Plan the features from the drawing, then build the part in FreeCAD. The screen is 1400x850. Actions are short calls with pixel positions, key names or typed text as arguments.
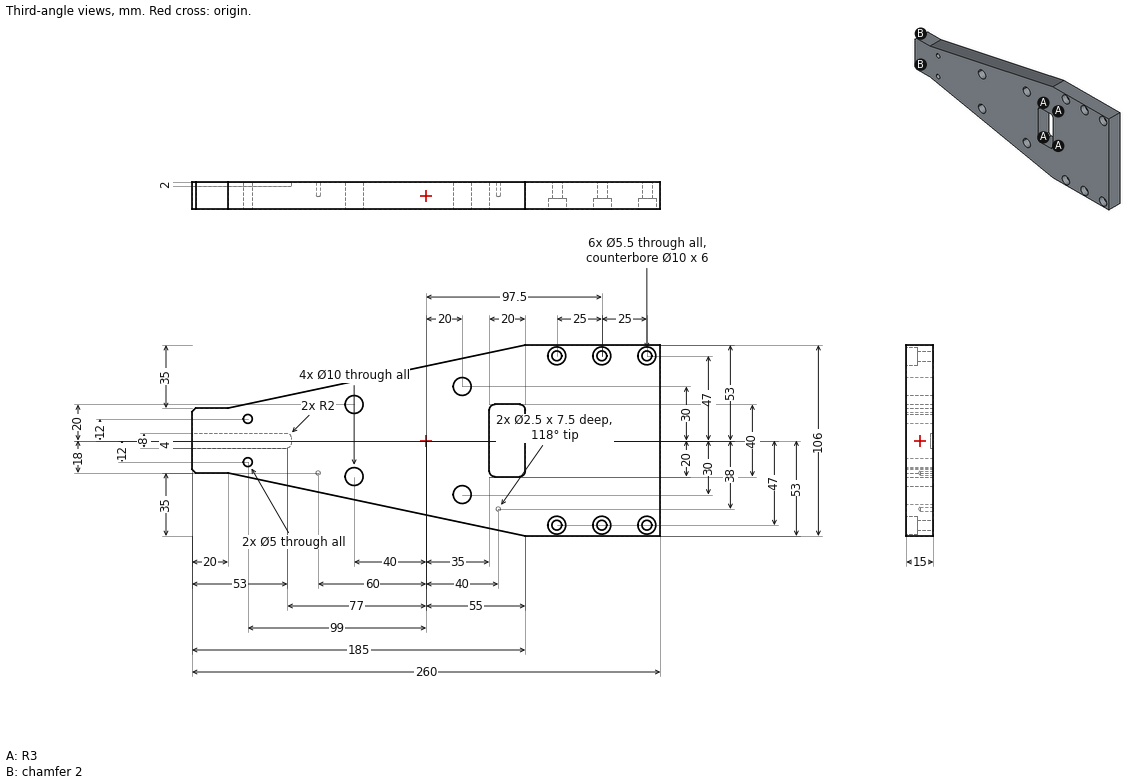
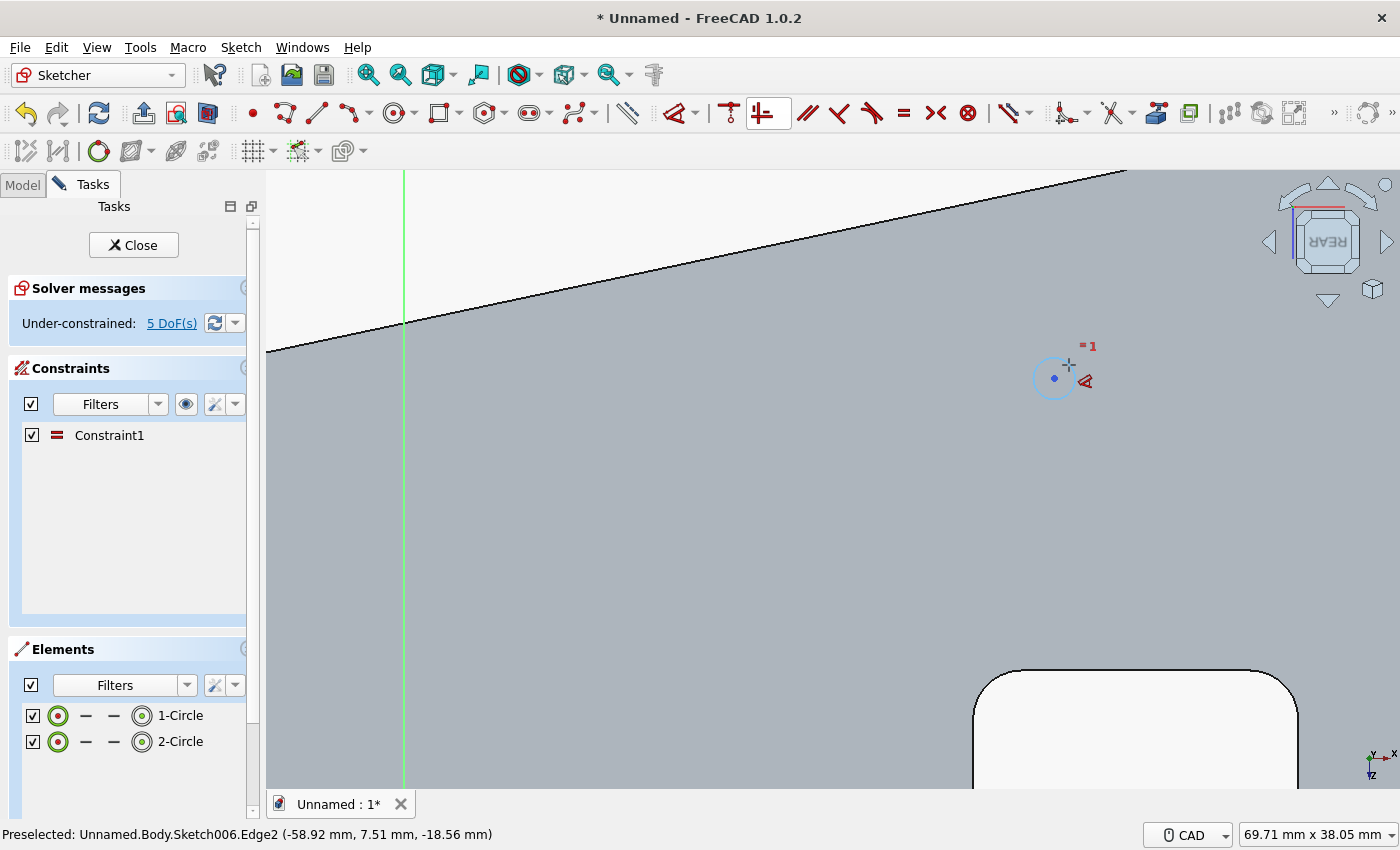
click(1069, 364)
click(1092, 341)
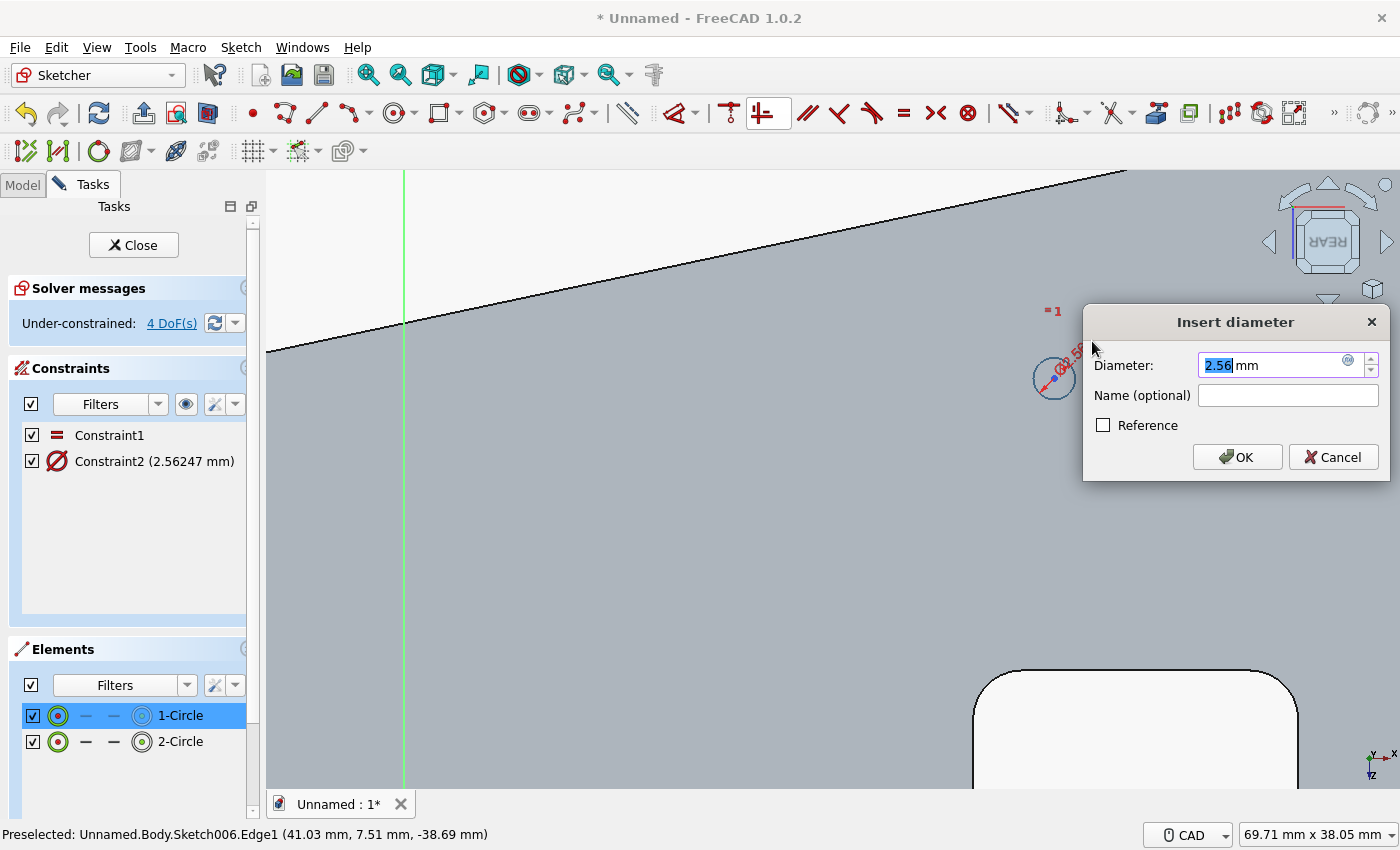
text(2.5)
key(Return)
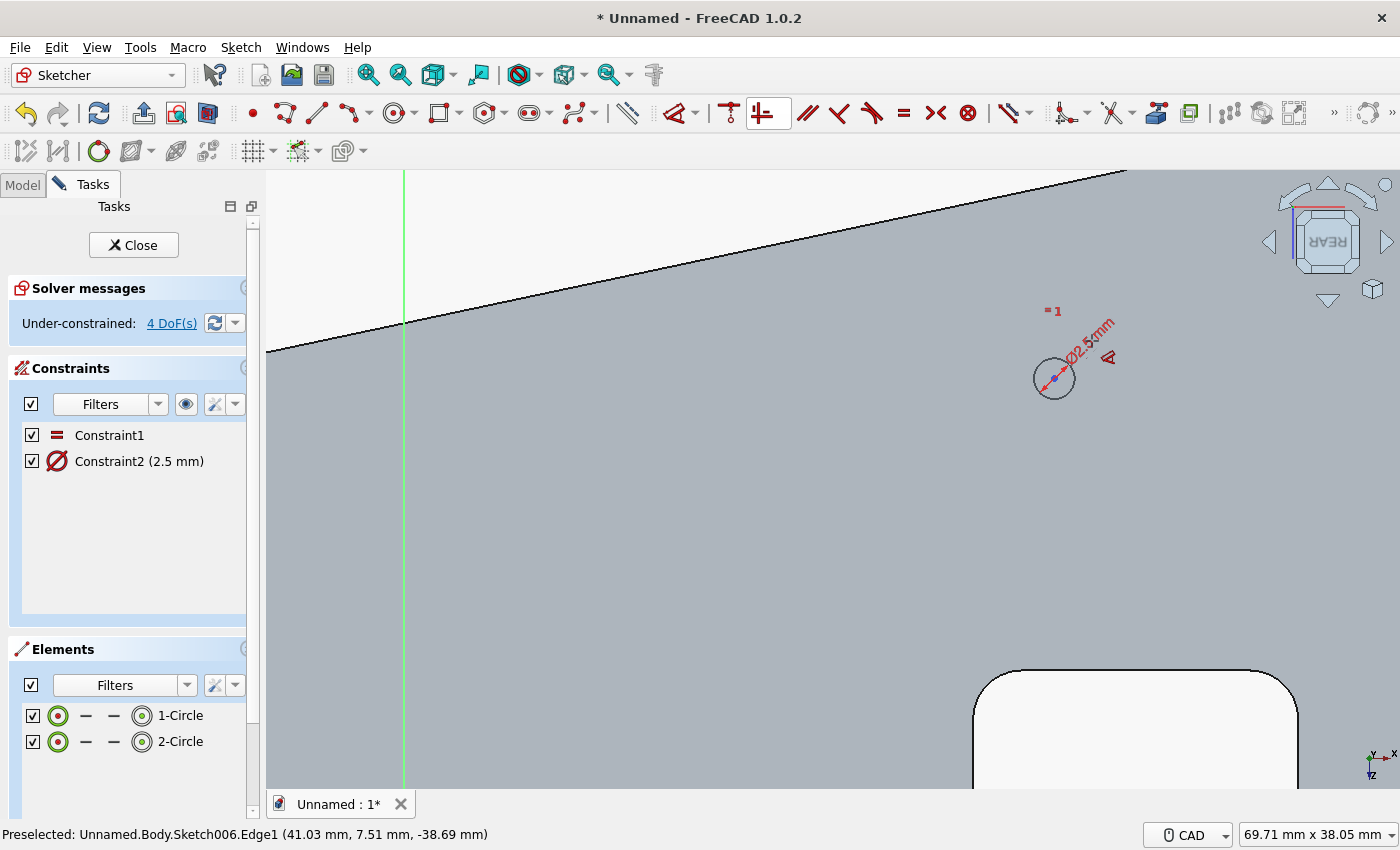
click(1054, 379)
click(729, 345)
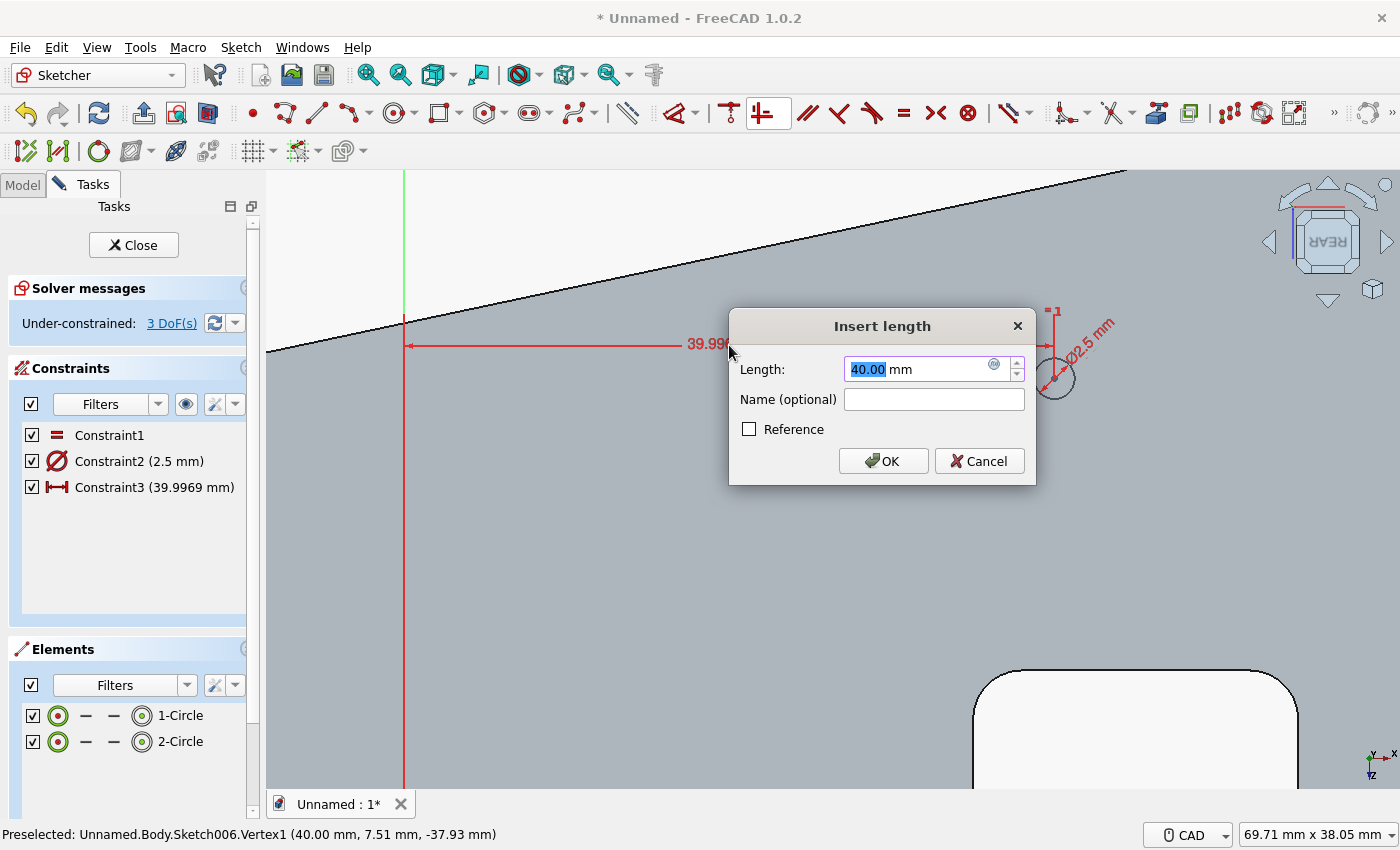
text(40)
key(Return)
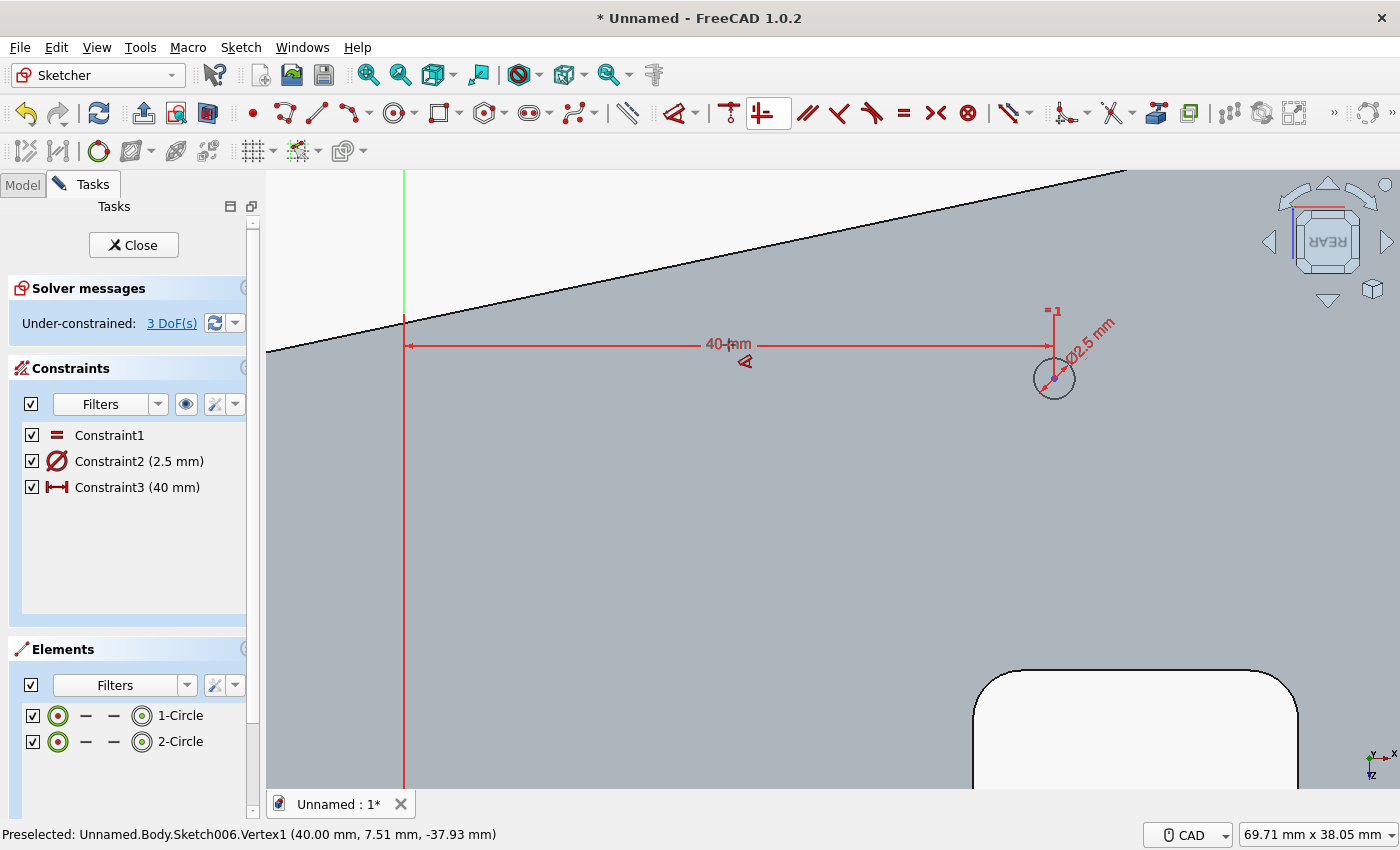
click(1054, 379)
click(1088, 570)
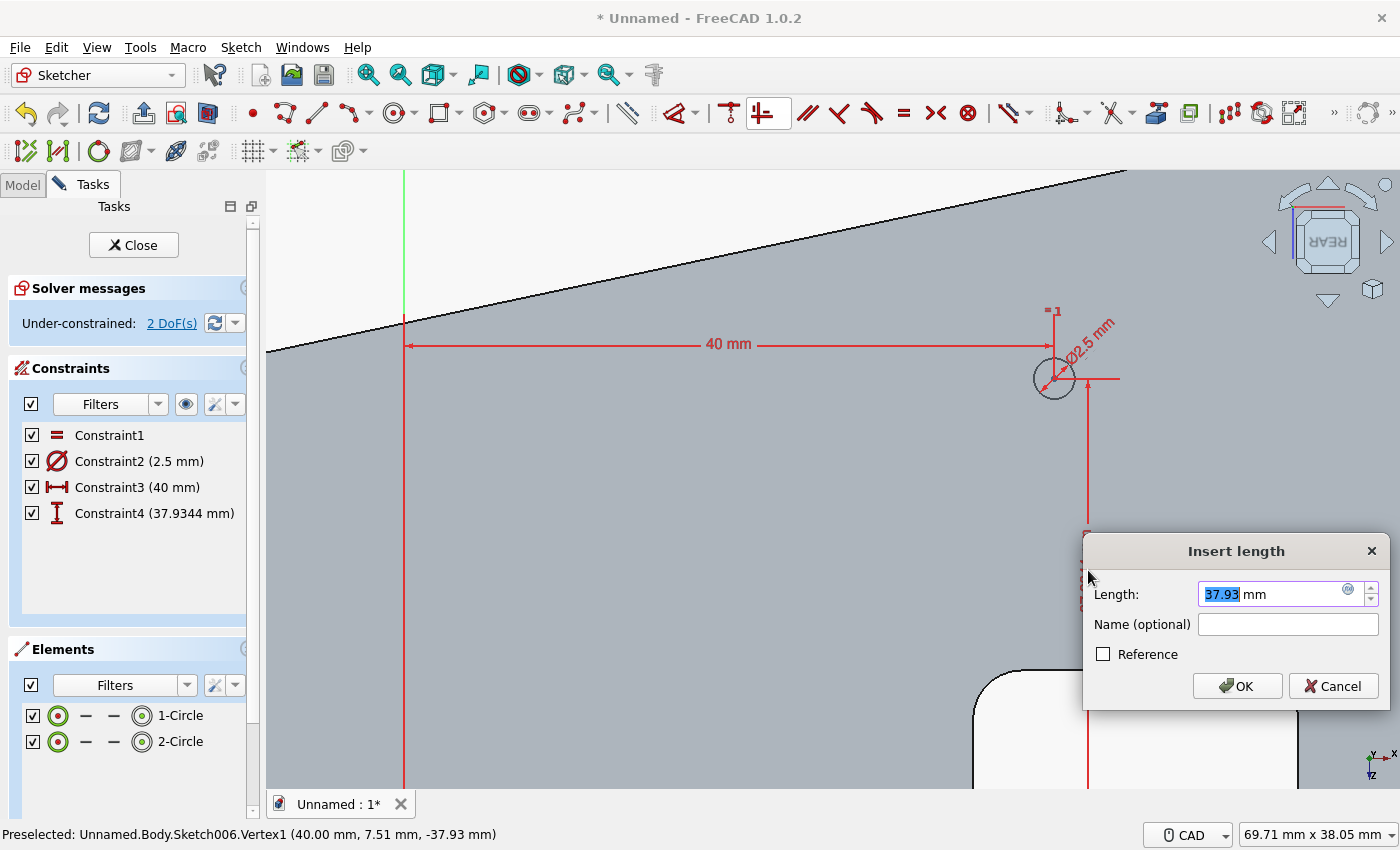
text(38)
key(Return)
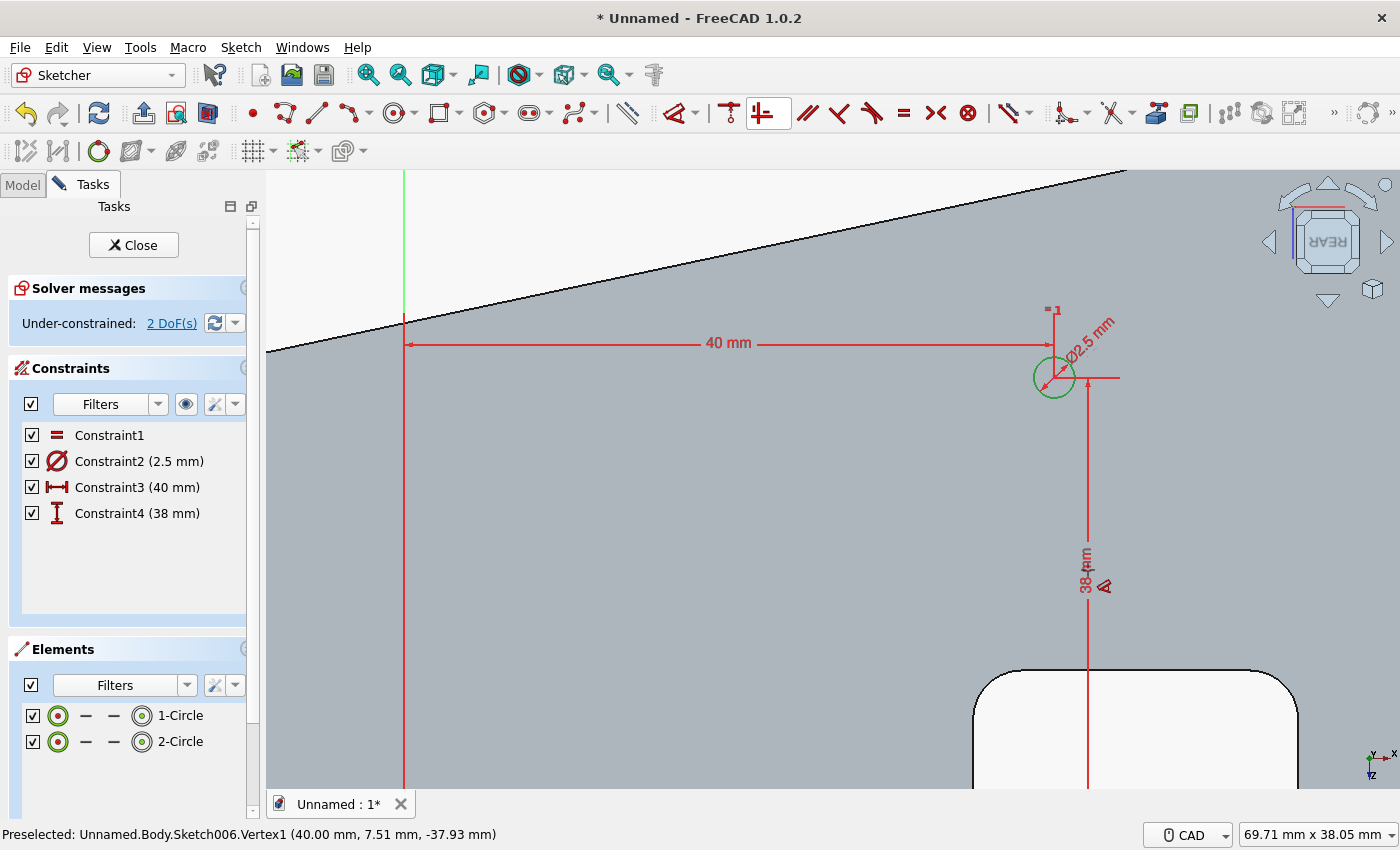
scroll(1069, 365, down, 5)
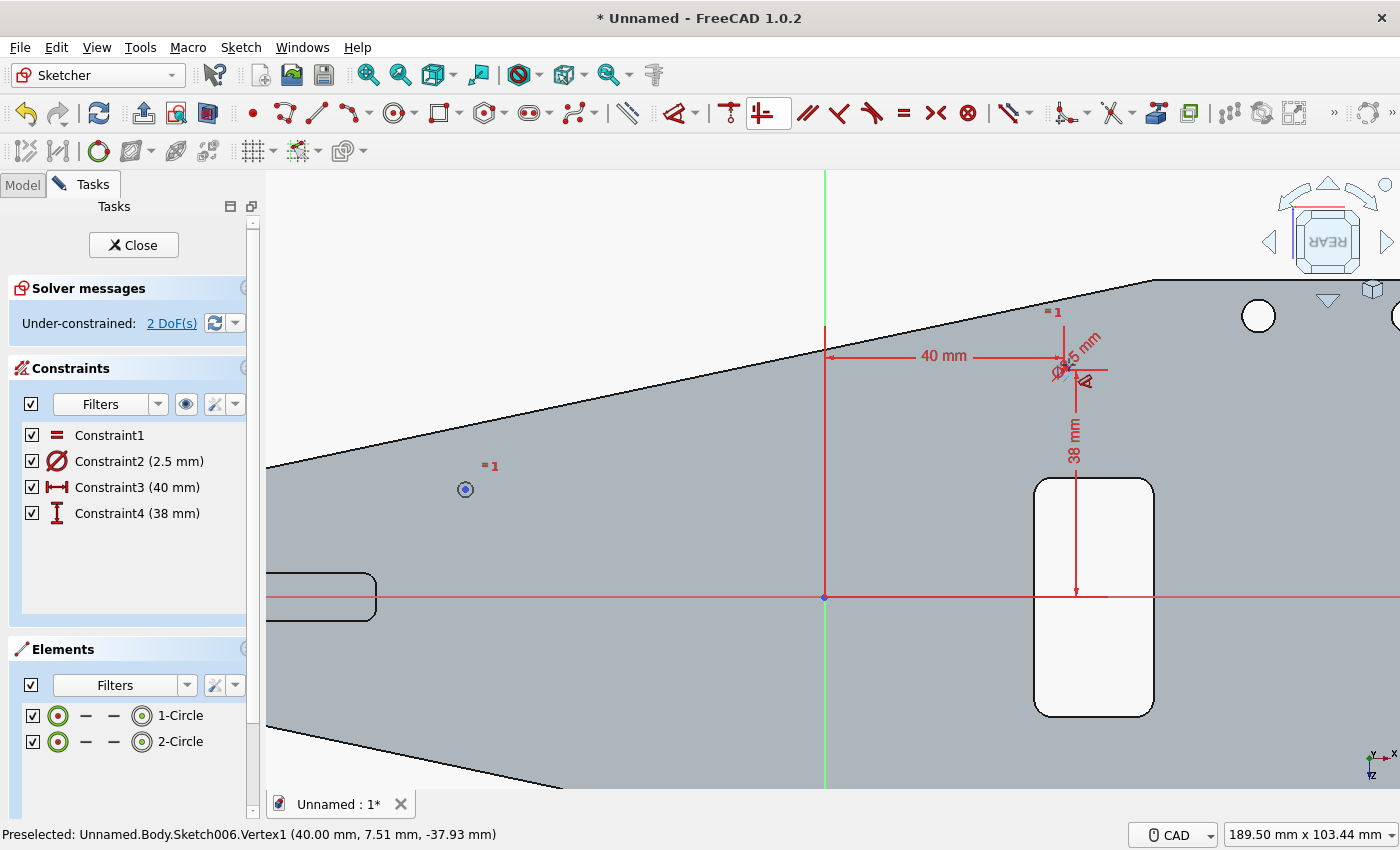
click(466, 490)
click(645, 631)